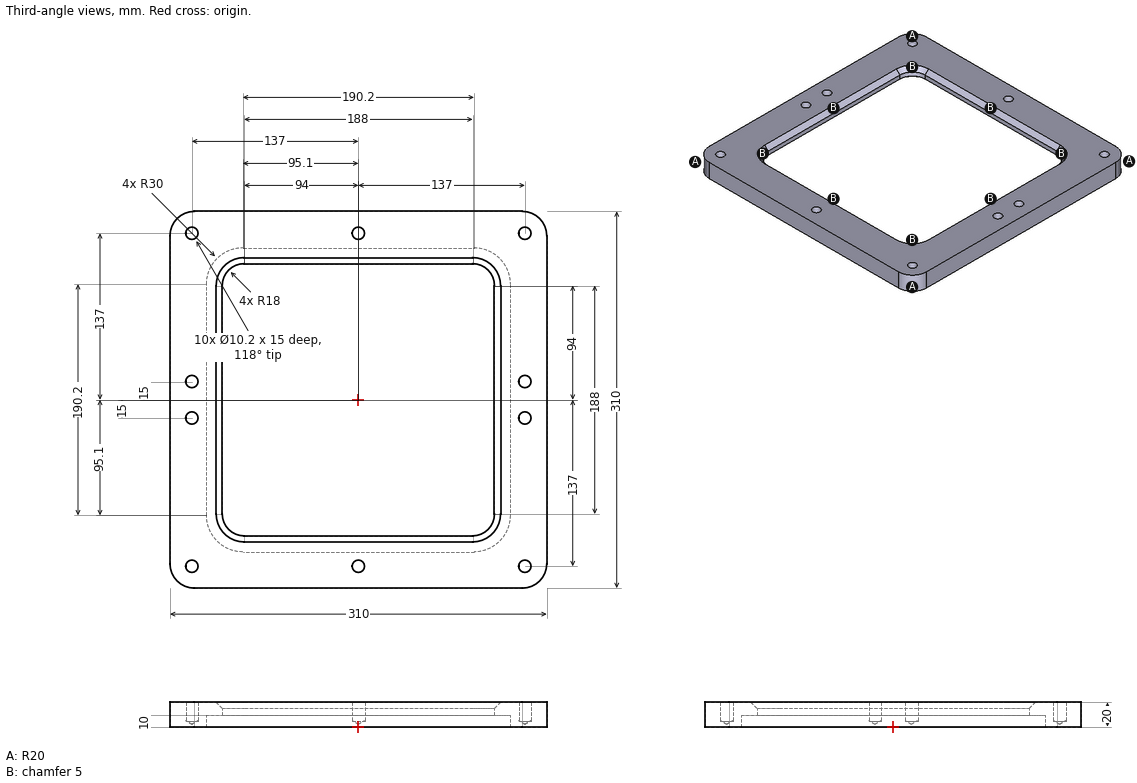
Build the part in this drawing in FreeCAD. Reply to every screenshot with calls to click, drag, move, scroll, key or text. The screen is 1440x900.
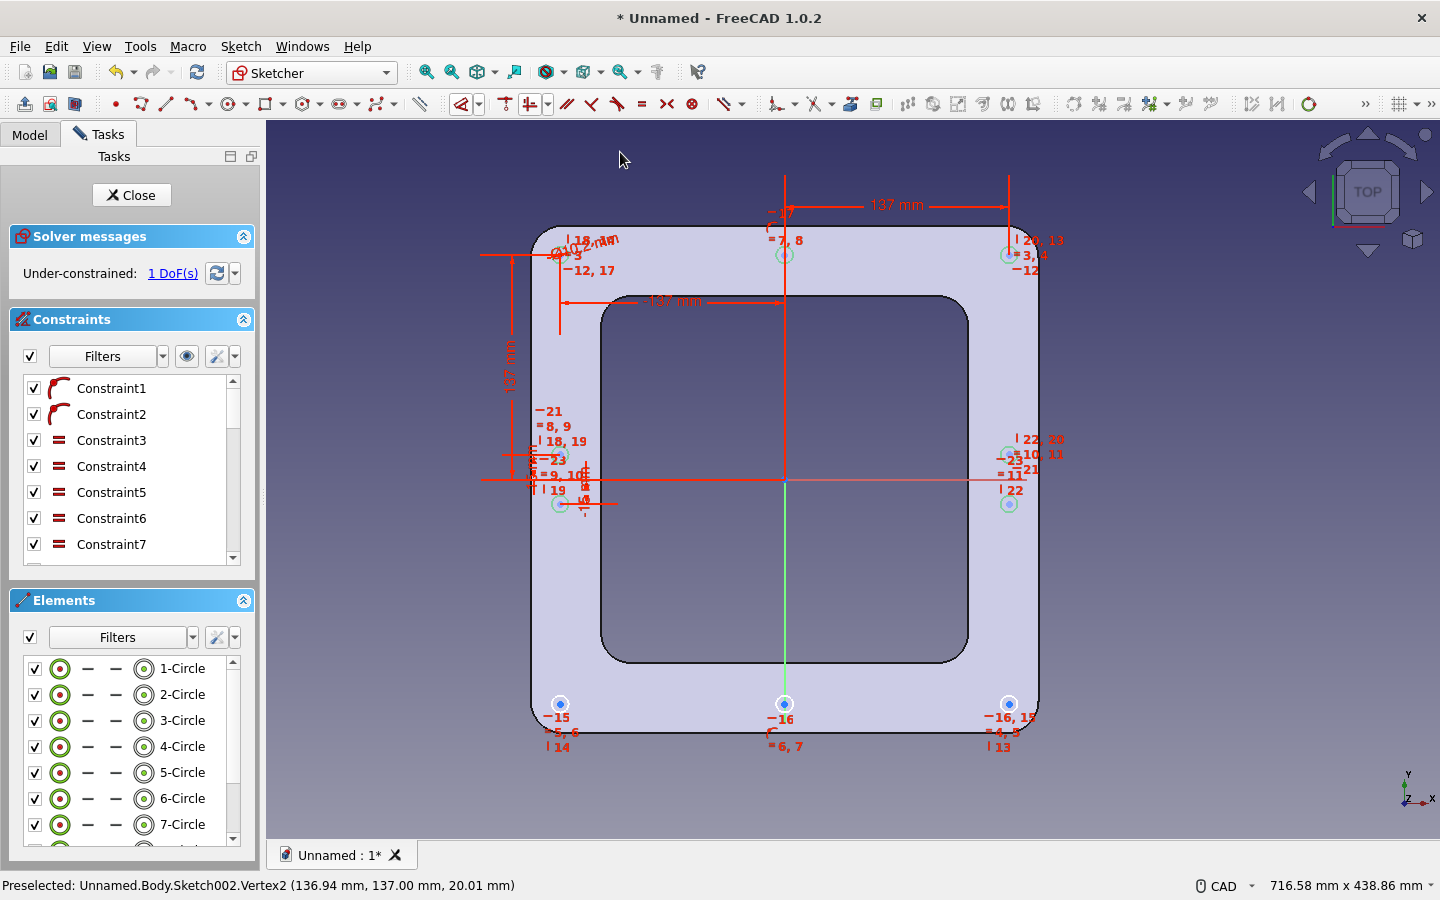
click(1009, 704)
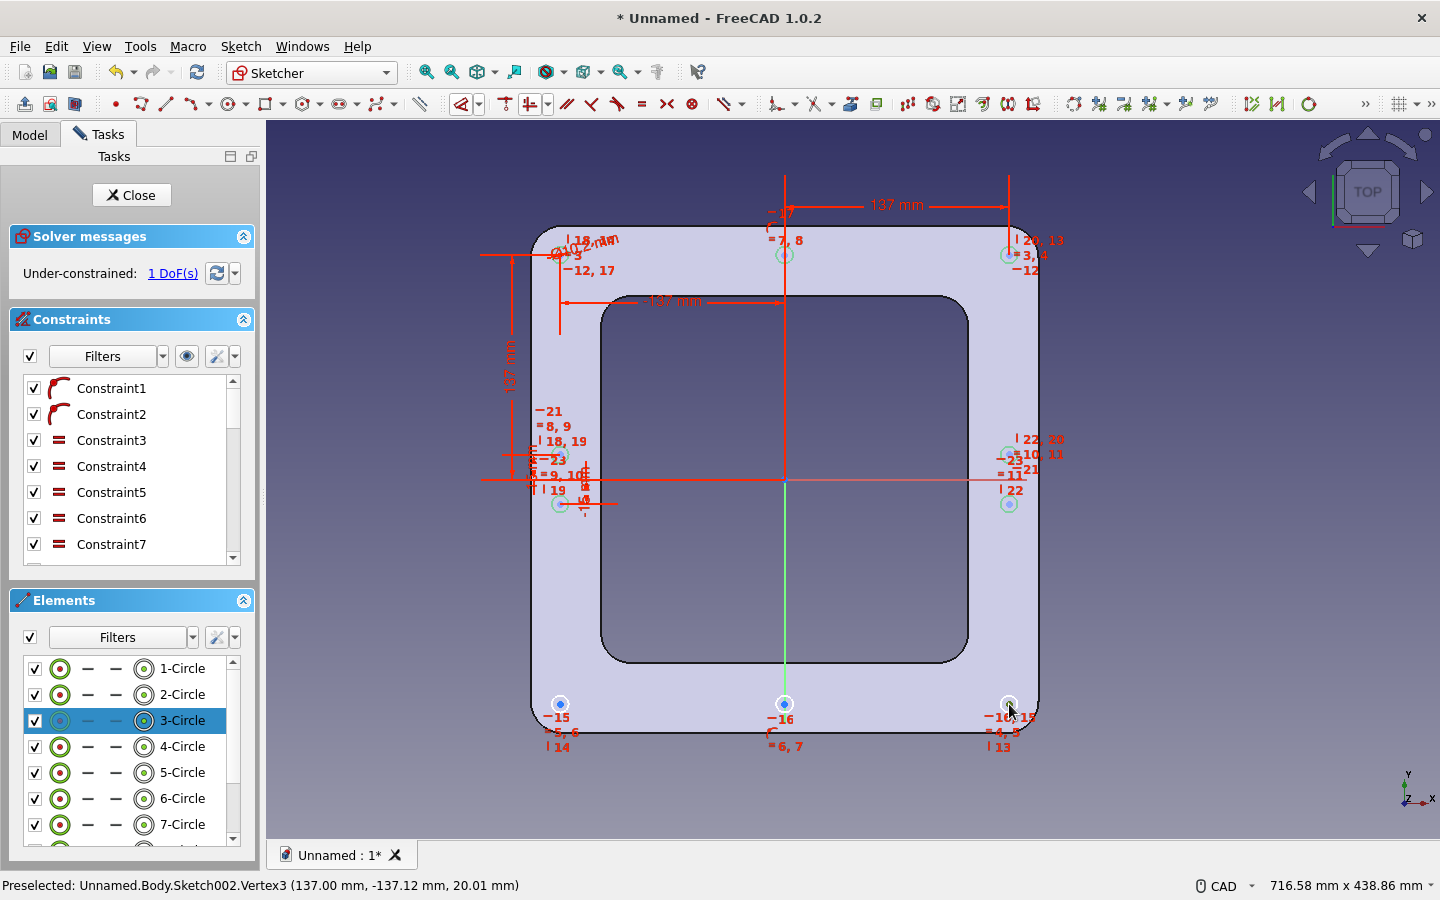
click(478, 104)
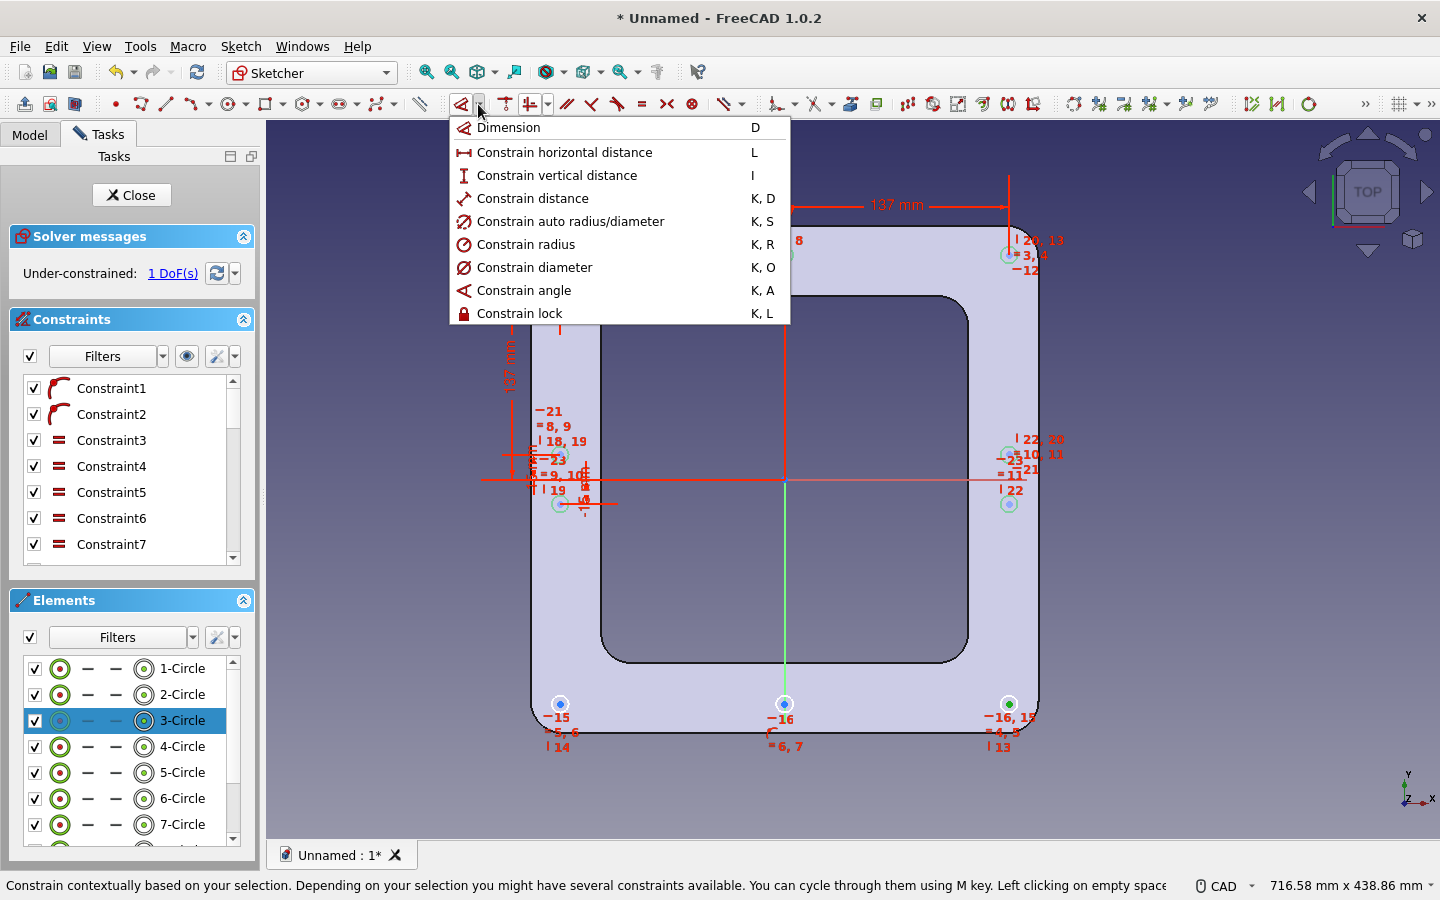
click(620, 176)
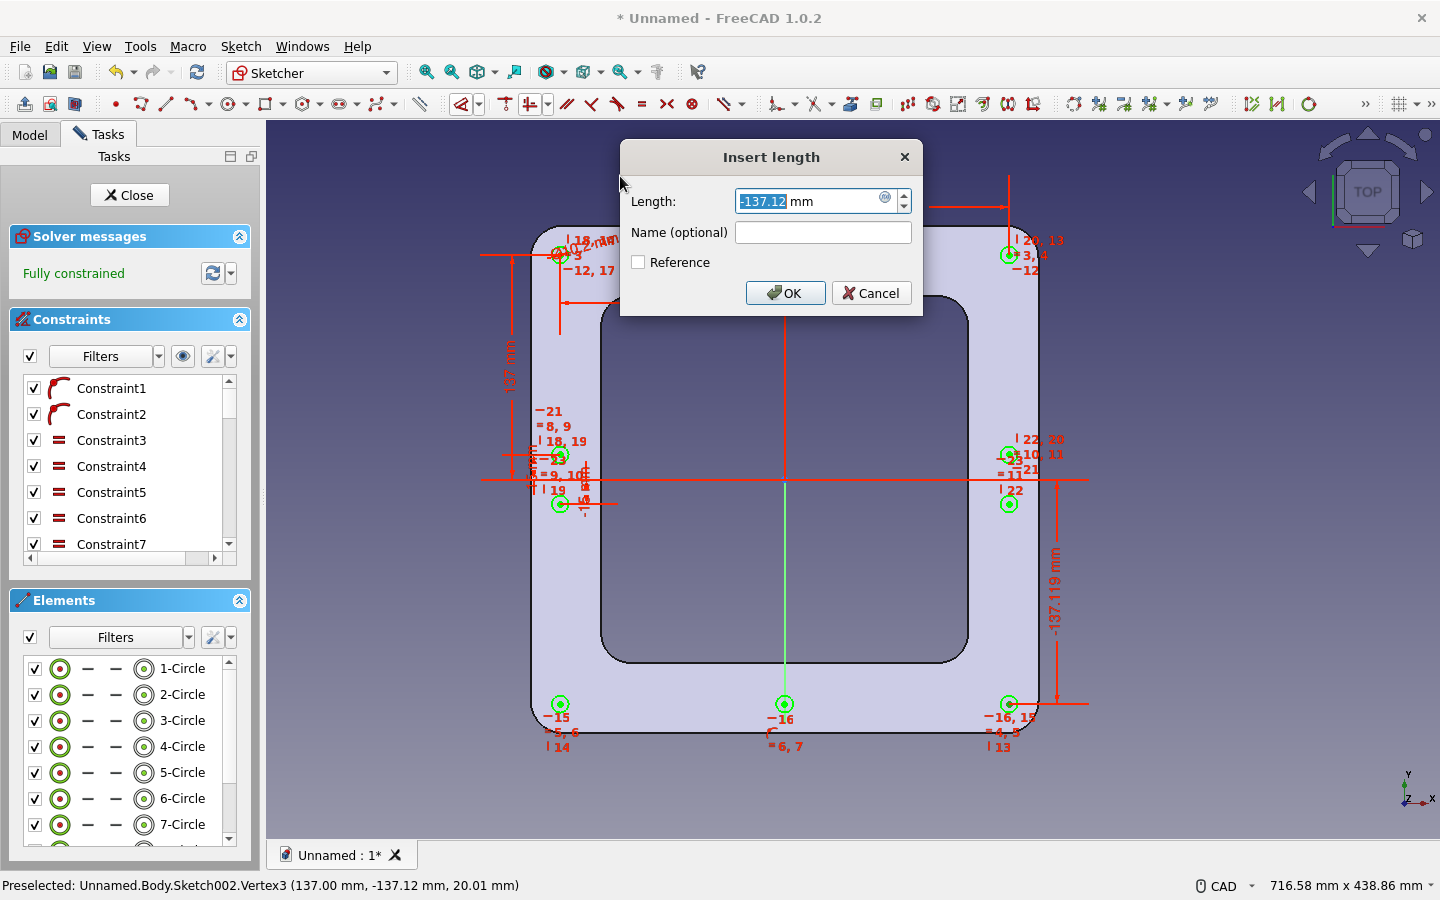
text(-137)
key(Return)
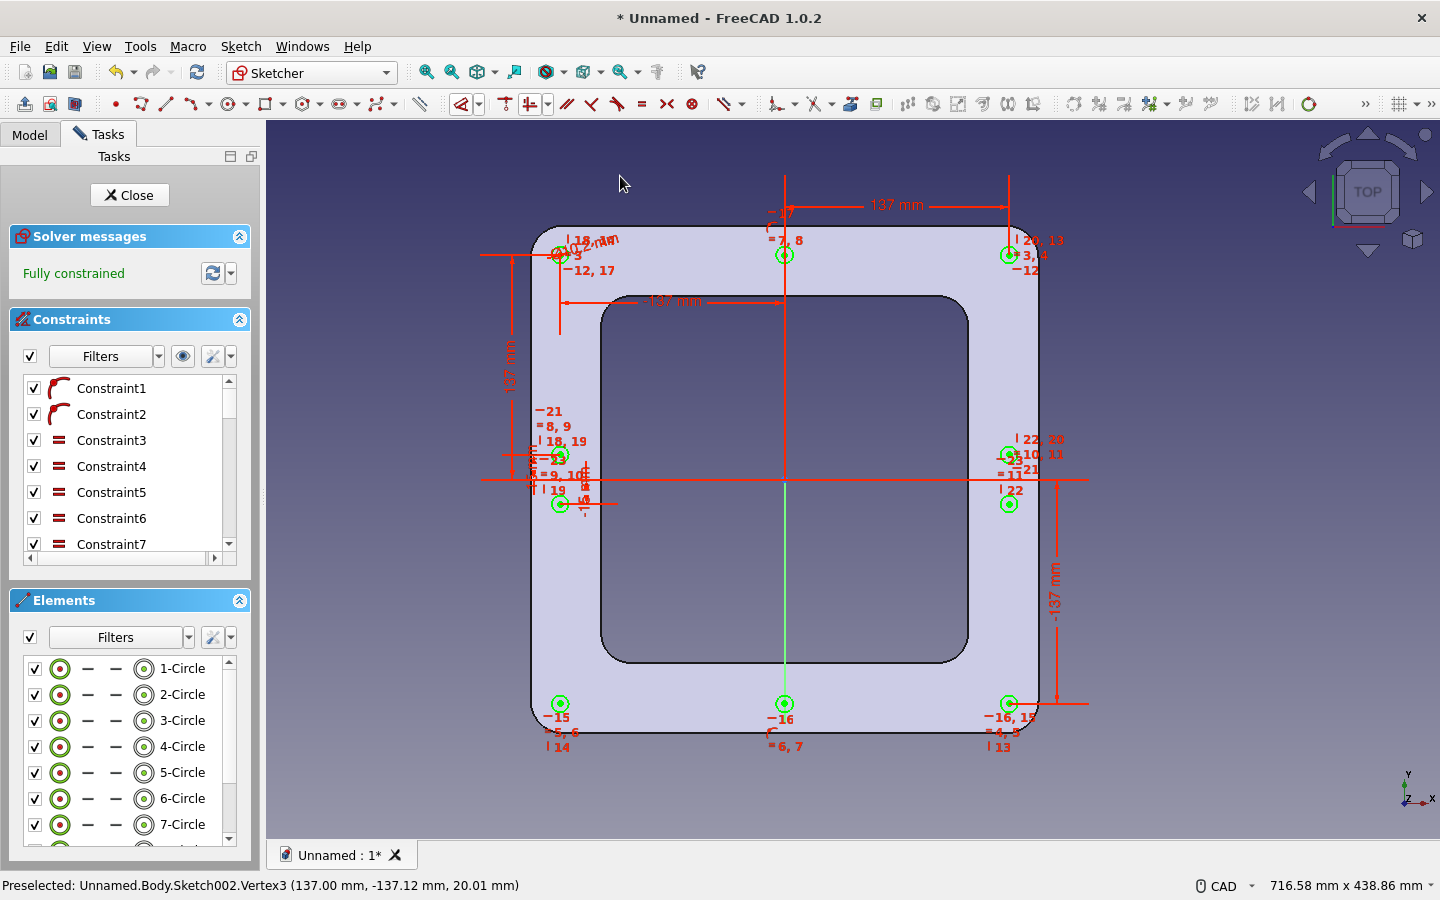
click(130, 195)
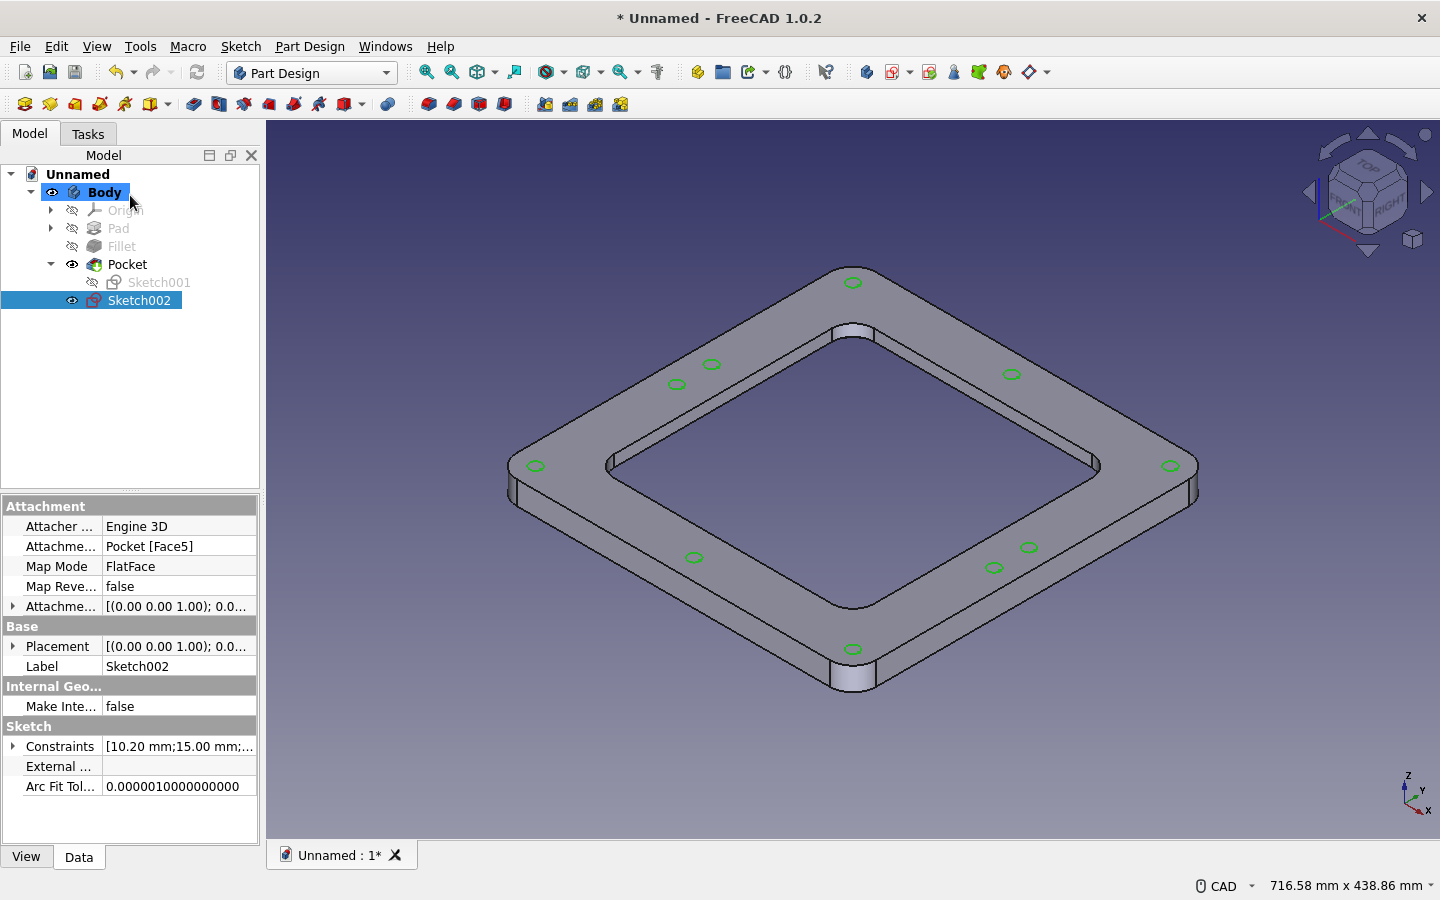
click(219, 104)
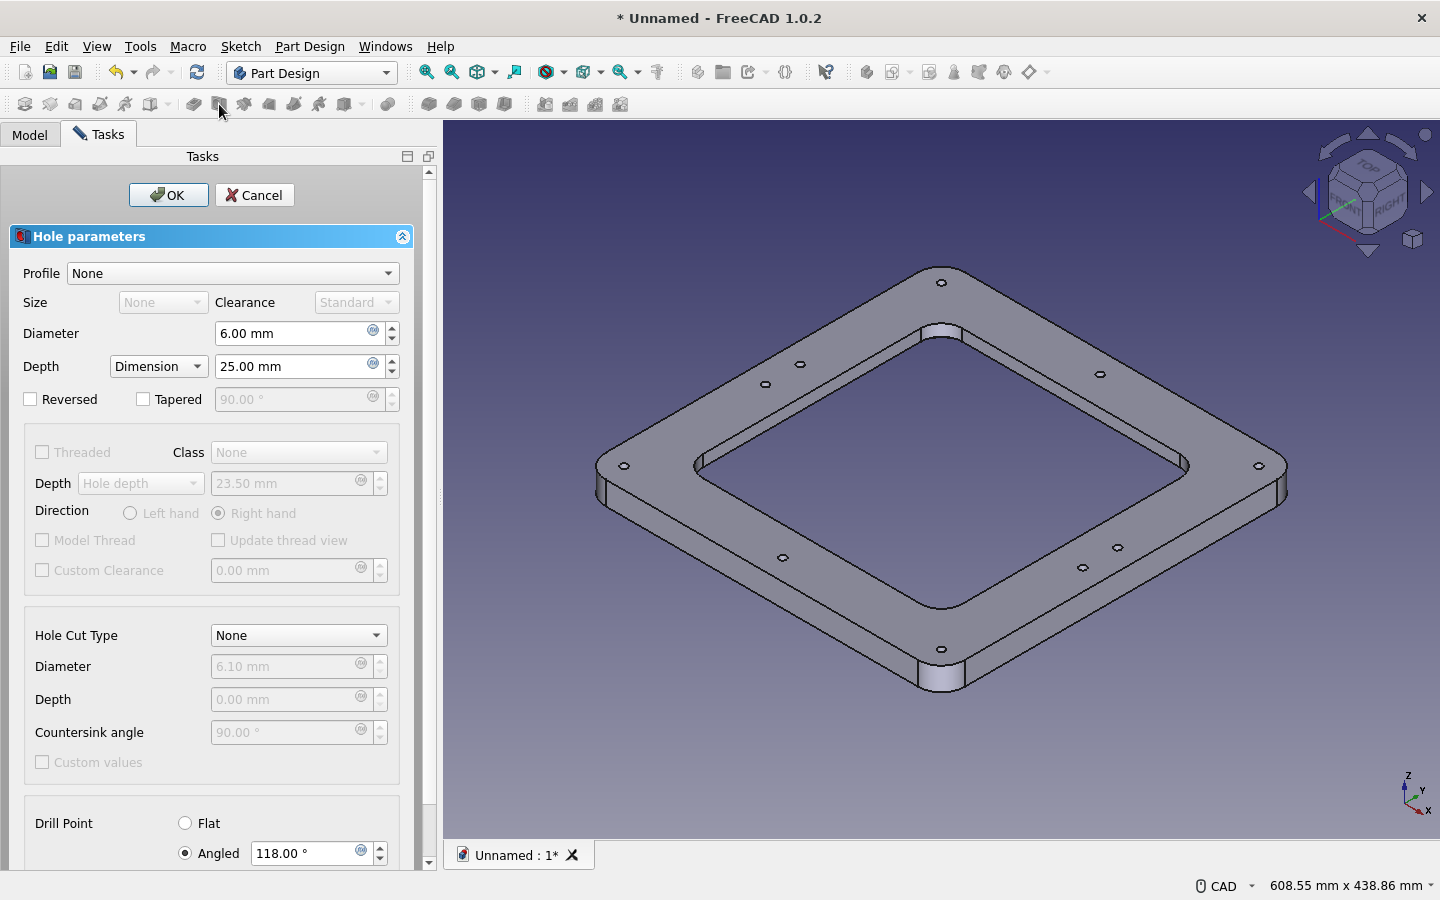
triple_click(300, 334)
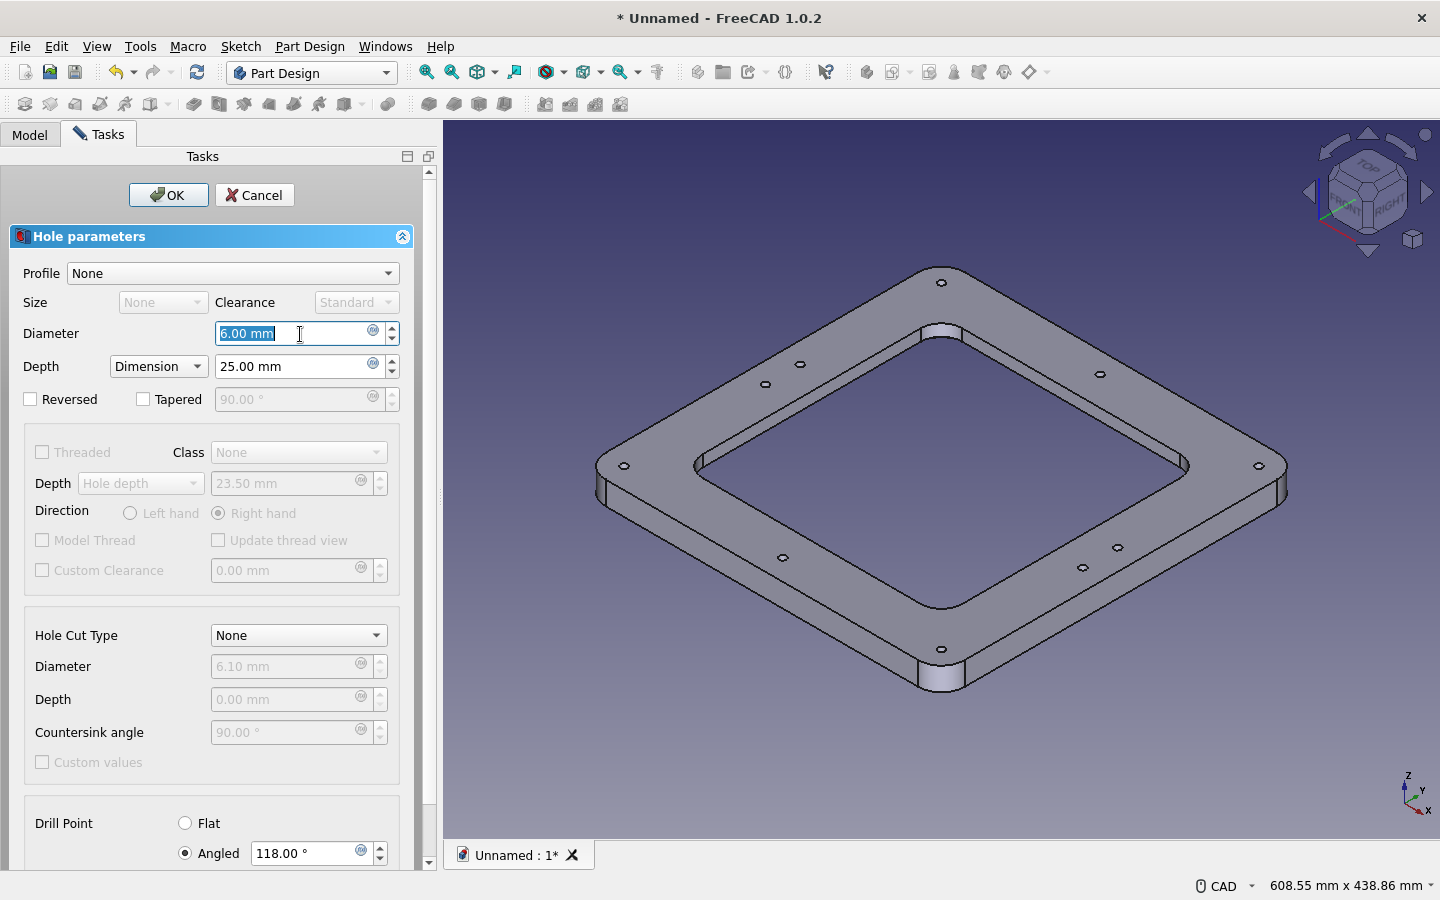
text(10.2)
key(Tab)